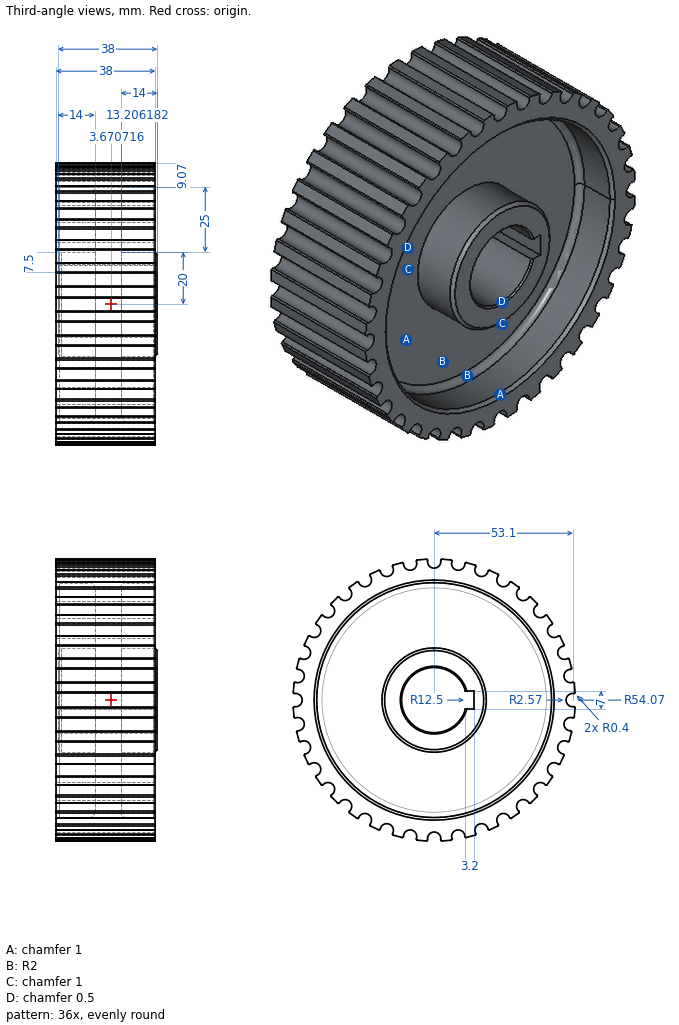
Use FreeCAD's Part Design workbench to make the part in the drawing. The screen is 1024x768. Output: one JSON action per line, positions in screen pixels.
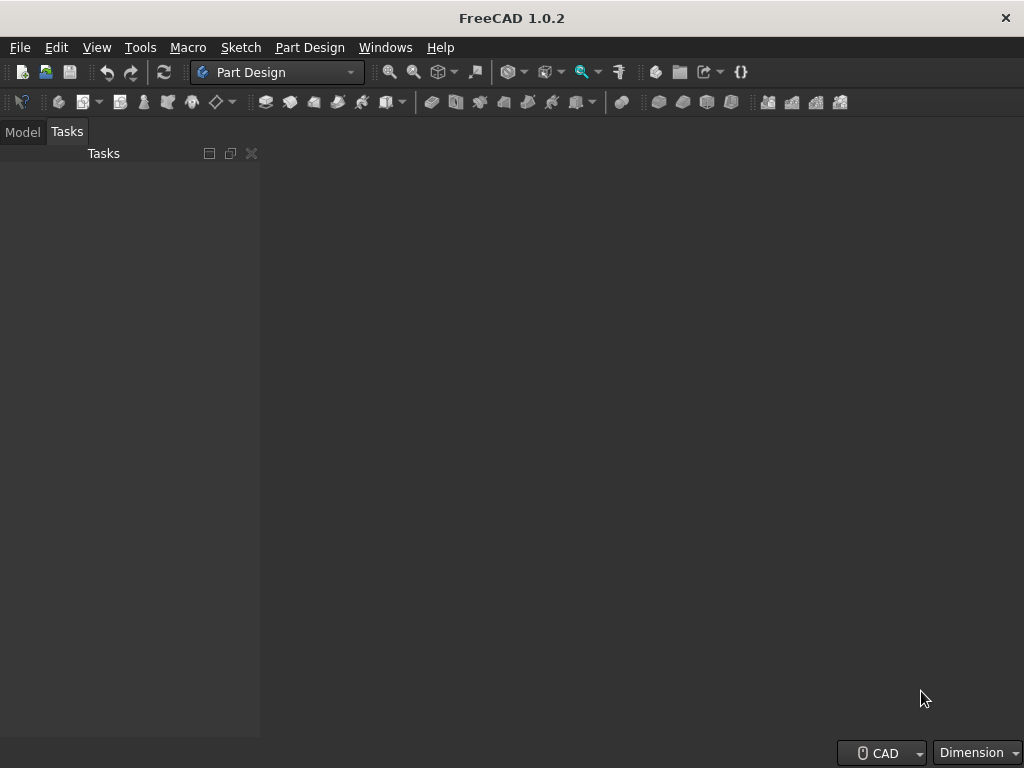
{"action": "left_click", "coordinate": [22, 72]}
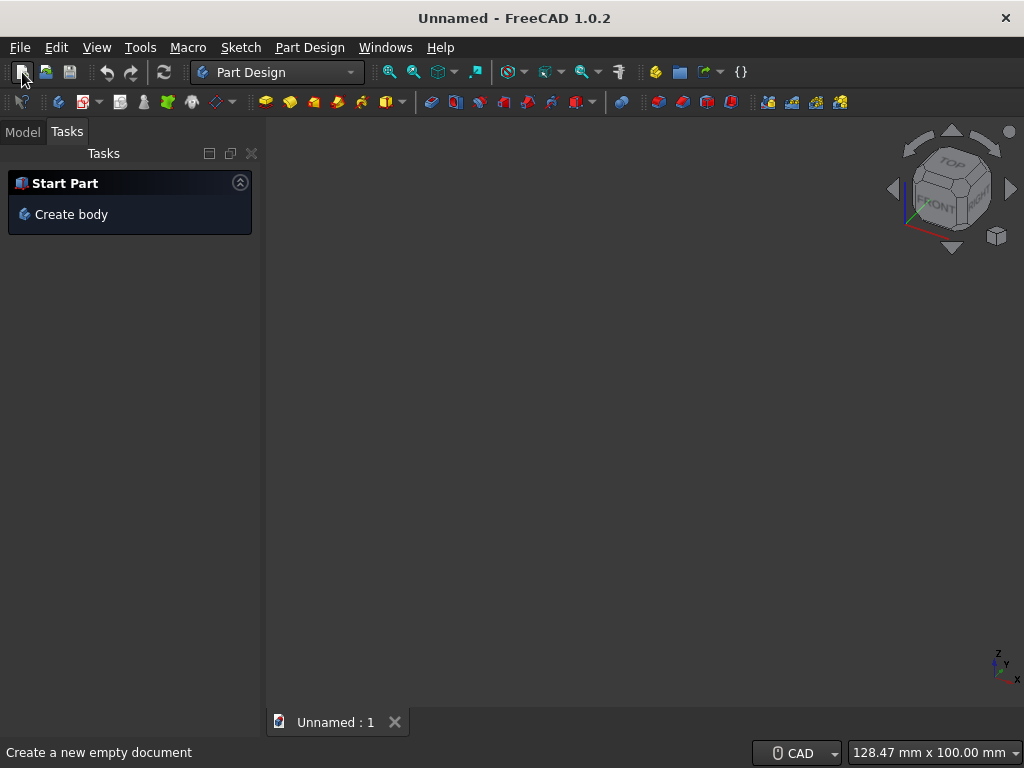
{"action": "left_click", "coordinate": [84, 102]}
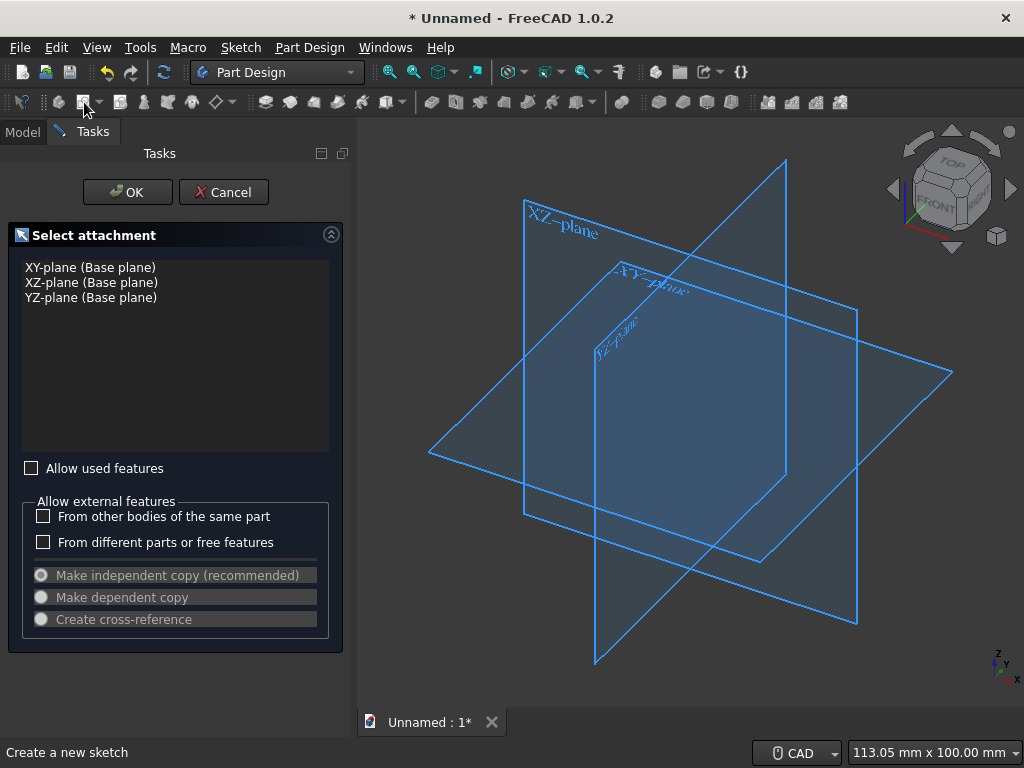
{"action": "left_click", "coordinate": [82, 268]}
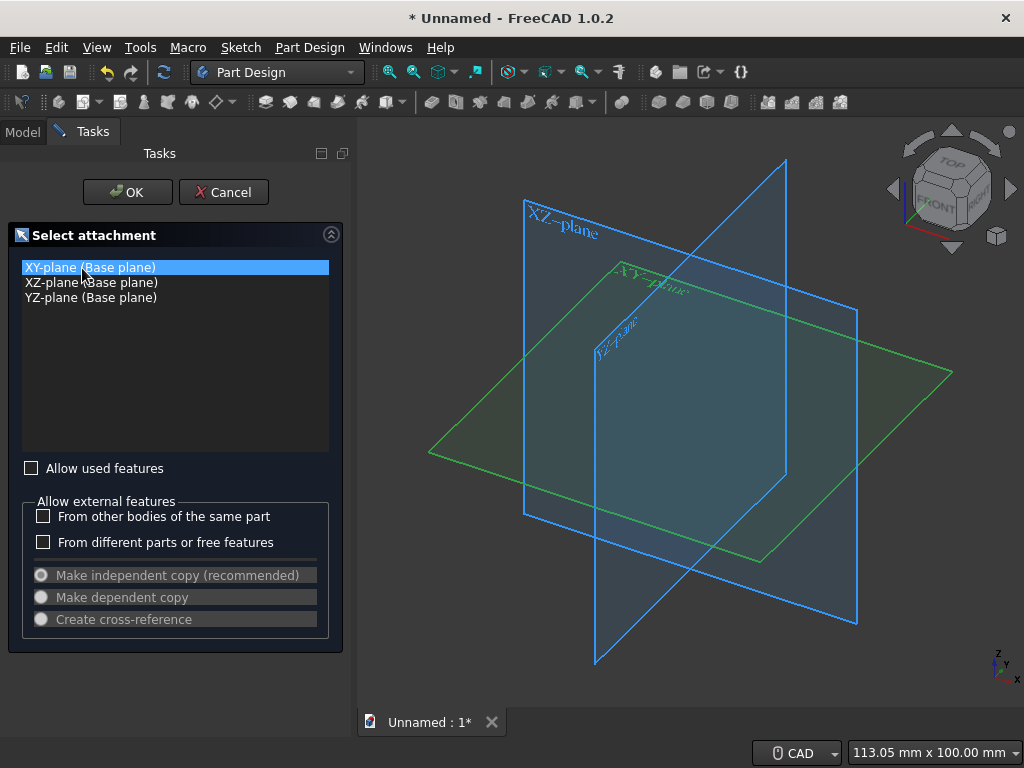
{"action": "left_click", "coordinate": [128, 192]}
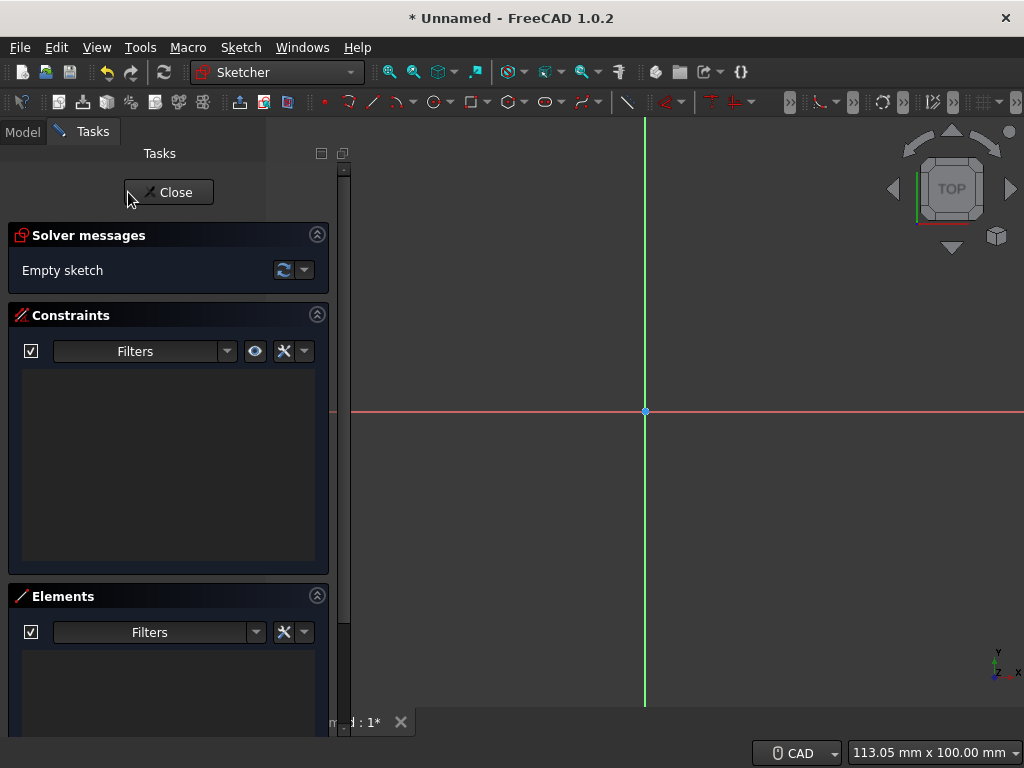
{"action": "scroll", "coordinate": [313, 679], "scroll_direction": "down", "scroll_amount": 1}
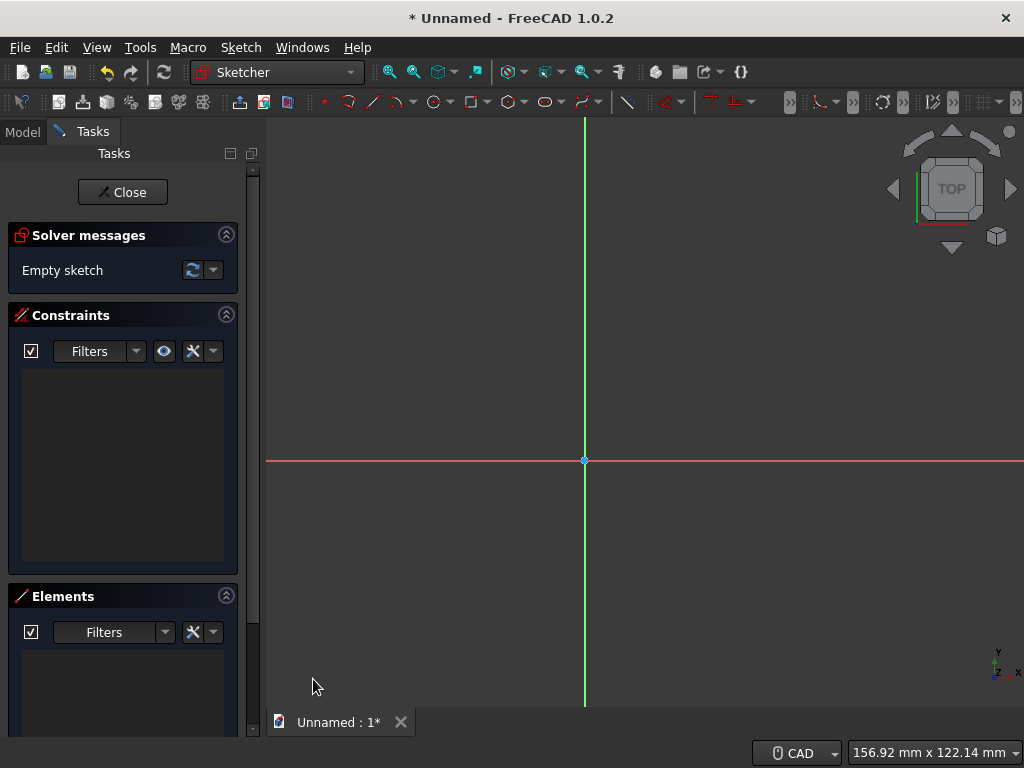
{"action": "scroll", "coordinate": [576, 163], "scroll_direction": "up", "scroll_amount": 2}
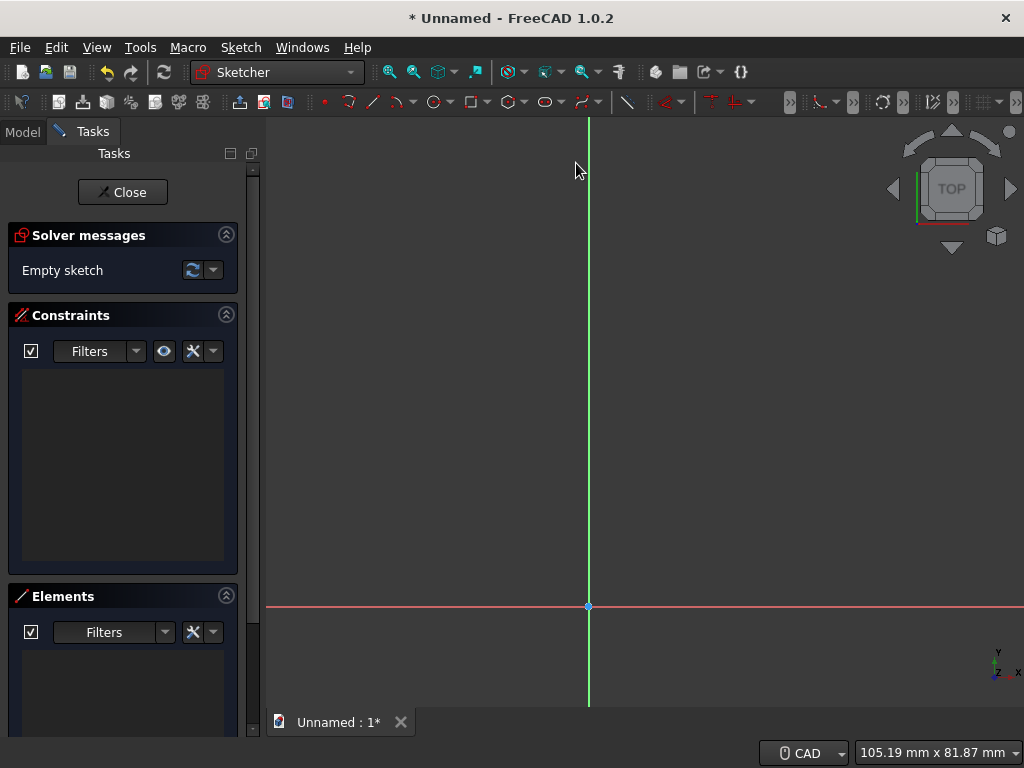
{"action": "left_click", "coordinate": [350, 102]}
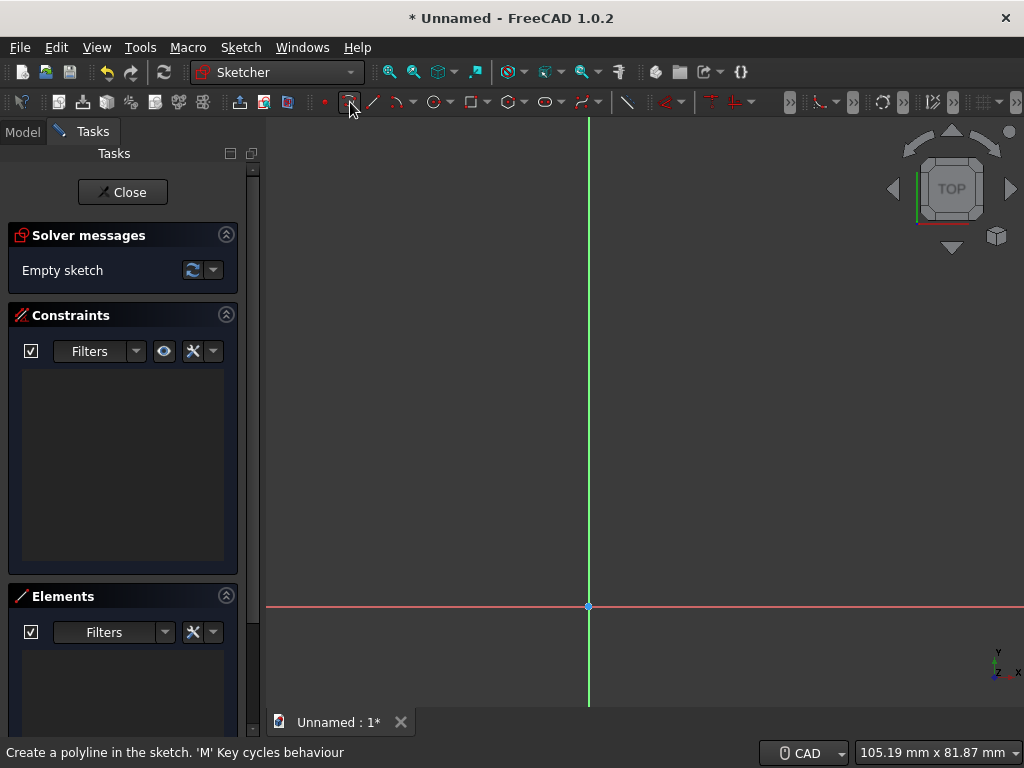
{"action": "left_click", "coordinate": [615, 463]}
{"action": "left_click", "coordinate": [615, 283]}
{"action": "left_click", "coordinate": [711, 283]}
{"action": "left_click", "coordinate": [711, 217]}
{"action": "left_click", "coordinate": [437, 217]}
{"action": "left_click", "coordinate": [437, 283]}
{"action": "left_click", "coordinate": [543, 283]}
{"action": "left_click", "coordinate": [543, 463]}
{"action": "left_click", "coordinate": [442, 463]}
{"action": "left_click", "coordinate": [442, 517]}
{"action": "left_click", "coordinate": [716, 517]}
{"action": "left_click", "coordinate": [716, 463]}
{"action": "left_click", "coordinate": [615, 464]}
{"action": "key", "text": "Escape"}
{"action": "key", "text": "Escape"}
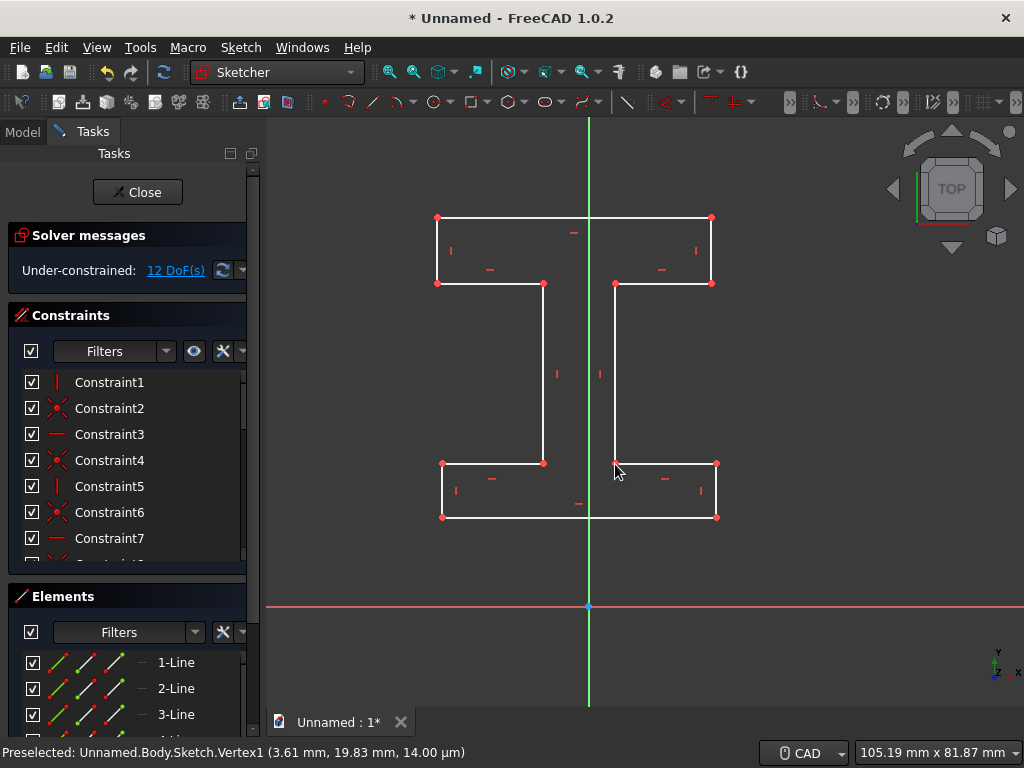
{"action": "left_click", "coordinate": [615, 410]}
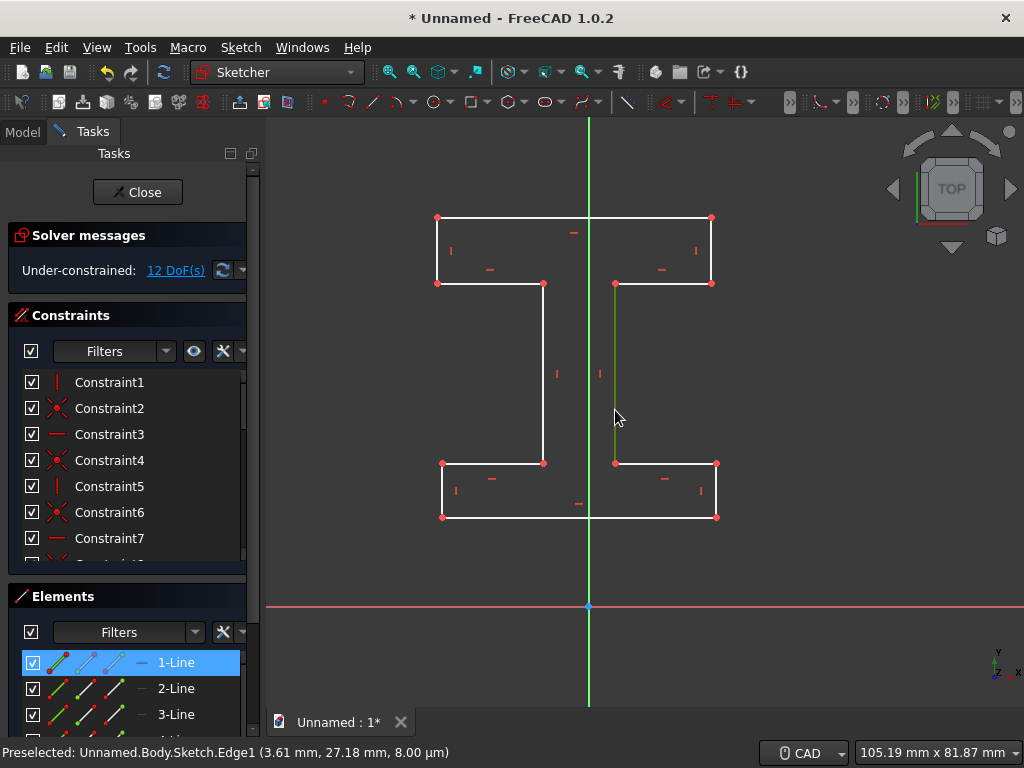
{"action": "left_click", "coordinate": [684, 102]}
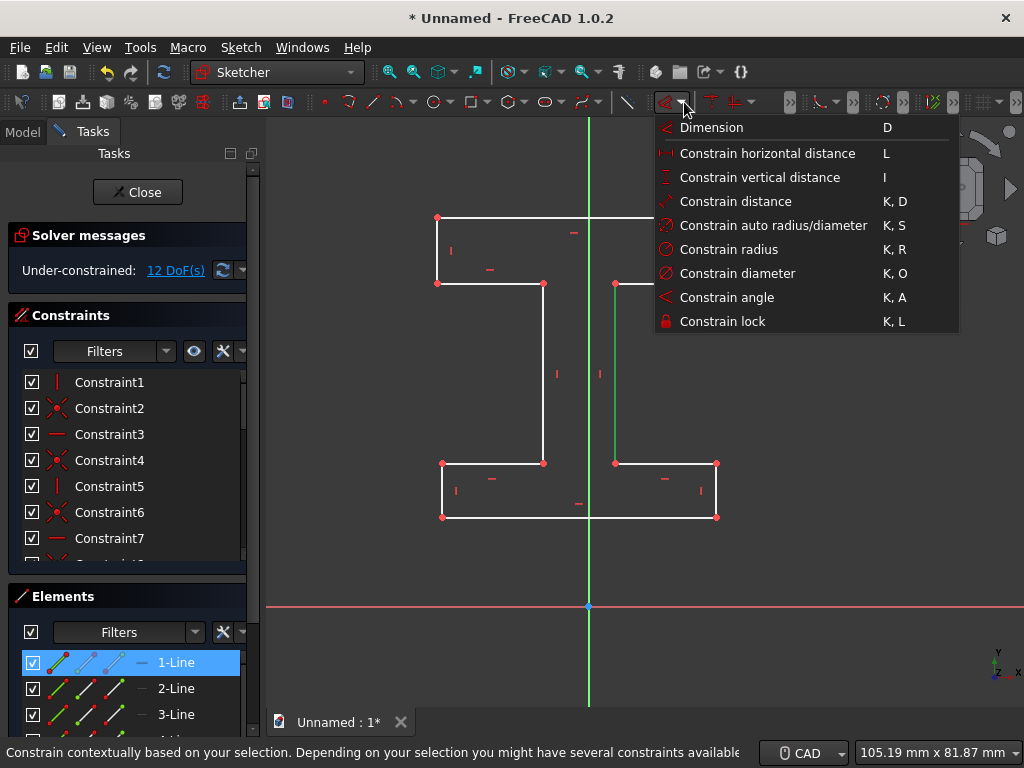
{"action": "left_click", "coordinate": [807, 177]}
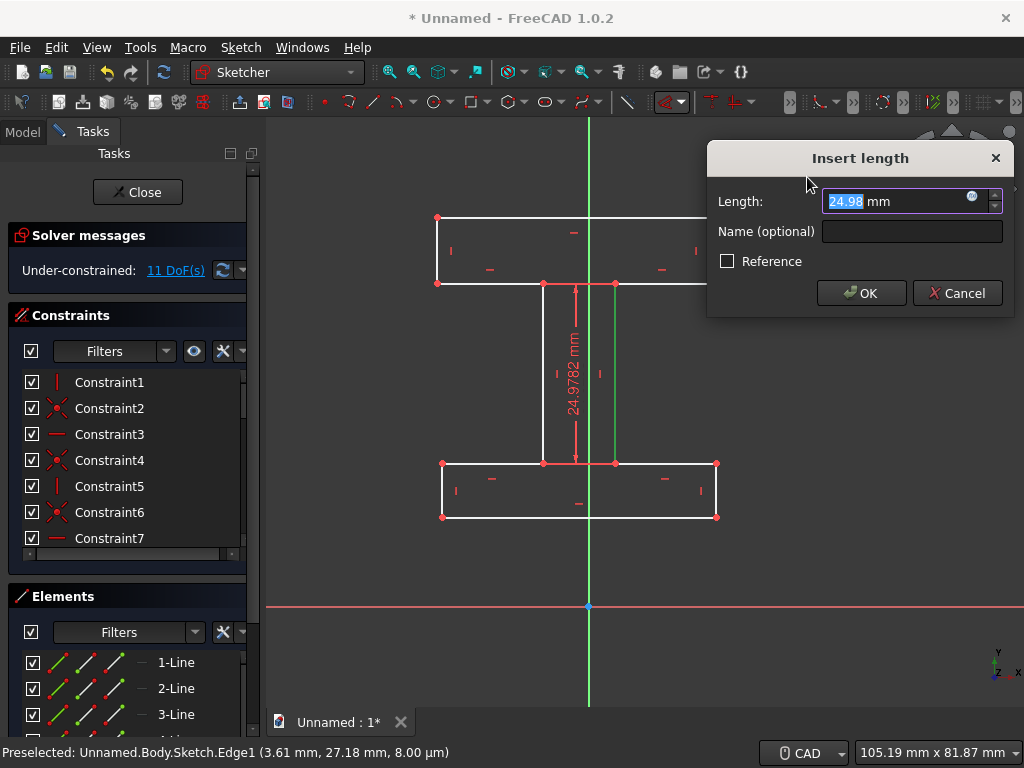
{"action": "type", "text": "25"}
{"action": "key", "text": "Return"}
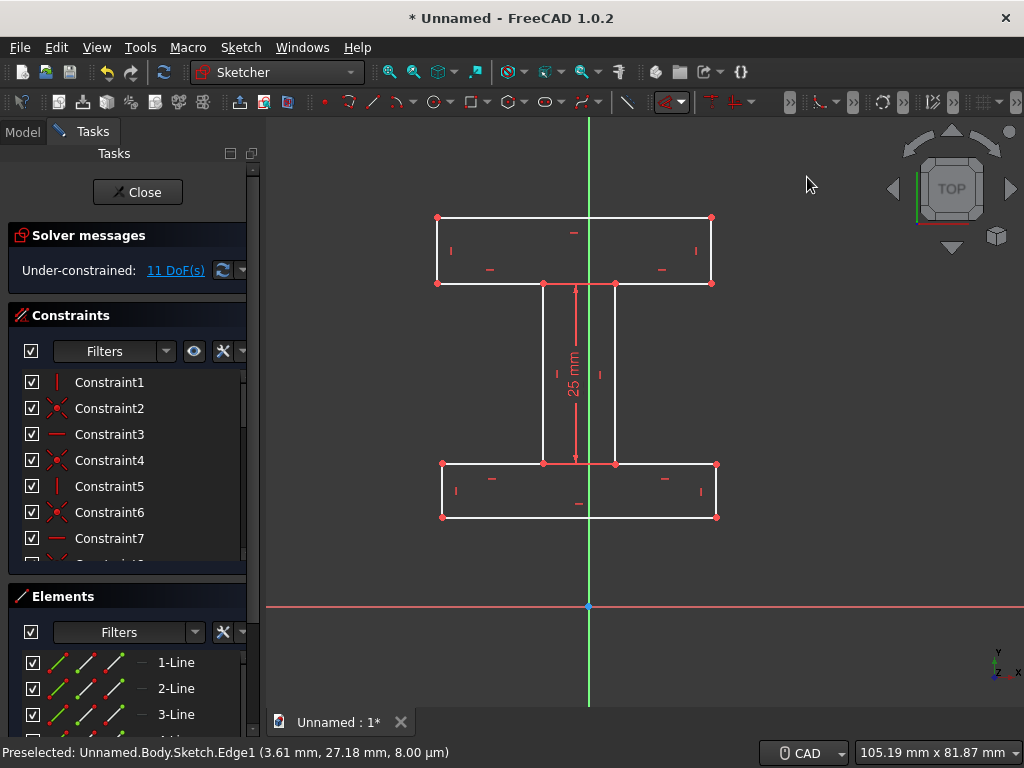
{"action": "left_click", "coordinate": [629, 218]}